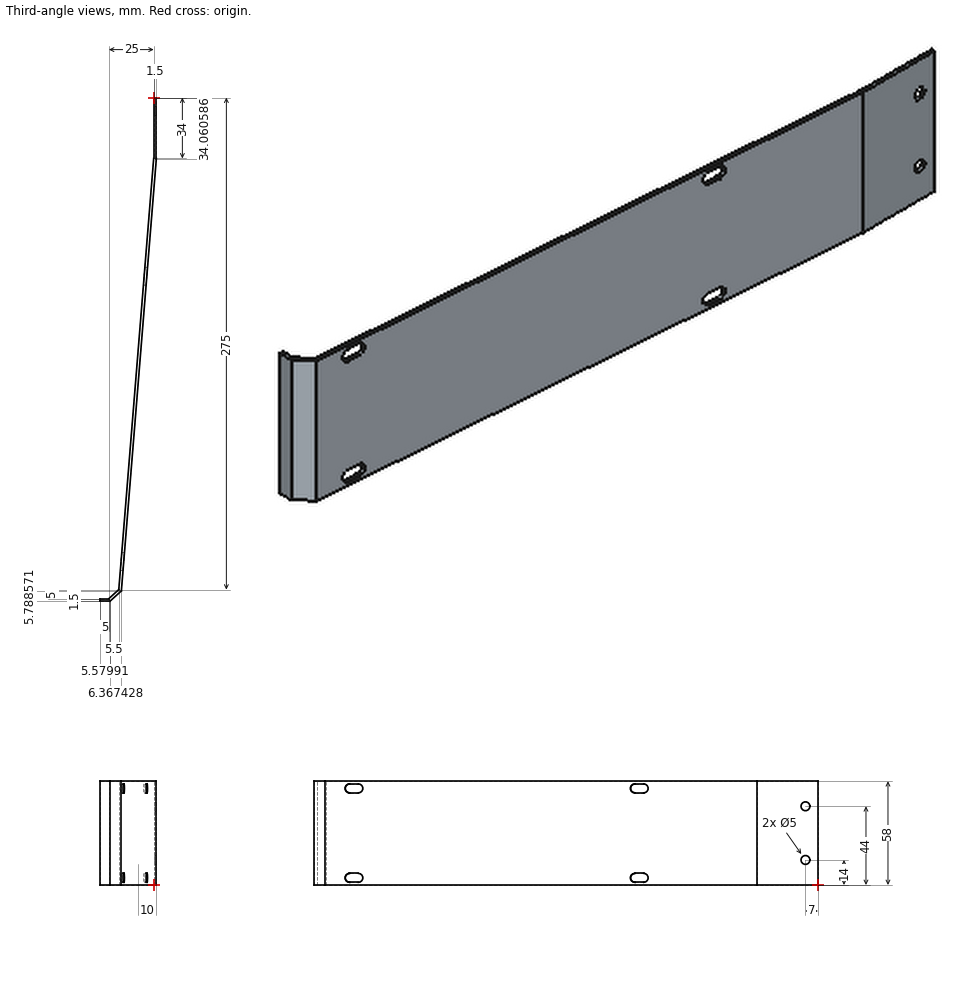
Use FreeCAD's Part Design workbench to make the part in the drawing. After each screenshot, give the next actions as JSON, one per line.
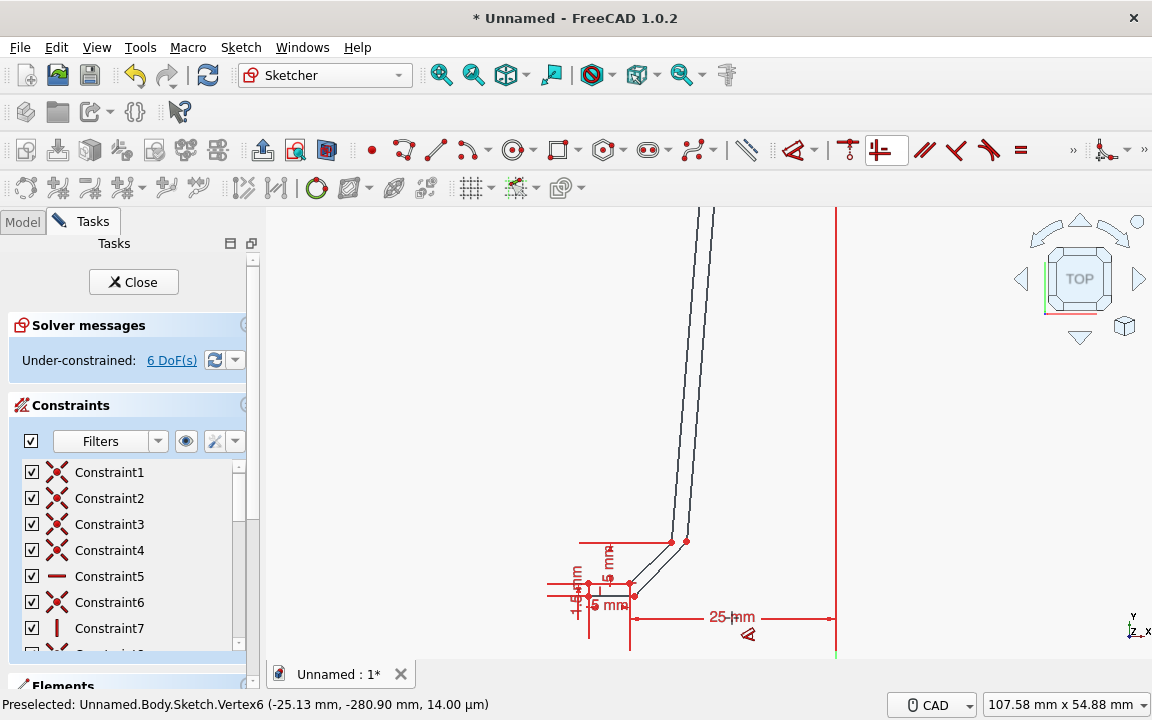
{"action": "left_click", "coordinate": [672, 543]}
{"action": "left_click", "coordinate": [870, 389]}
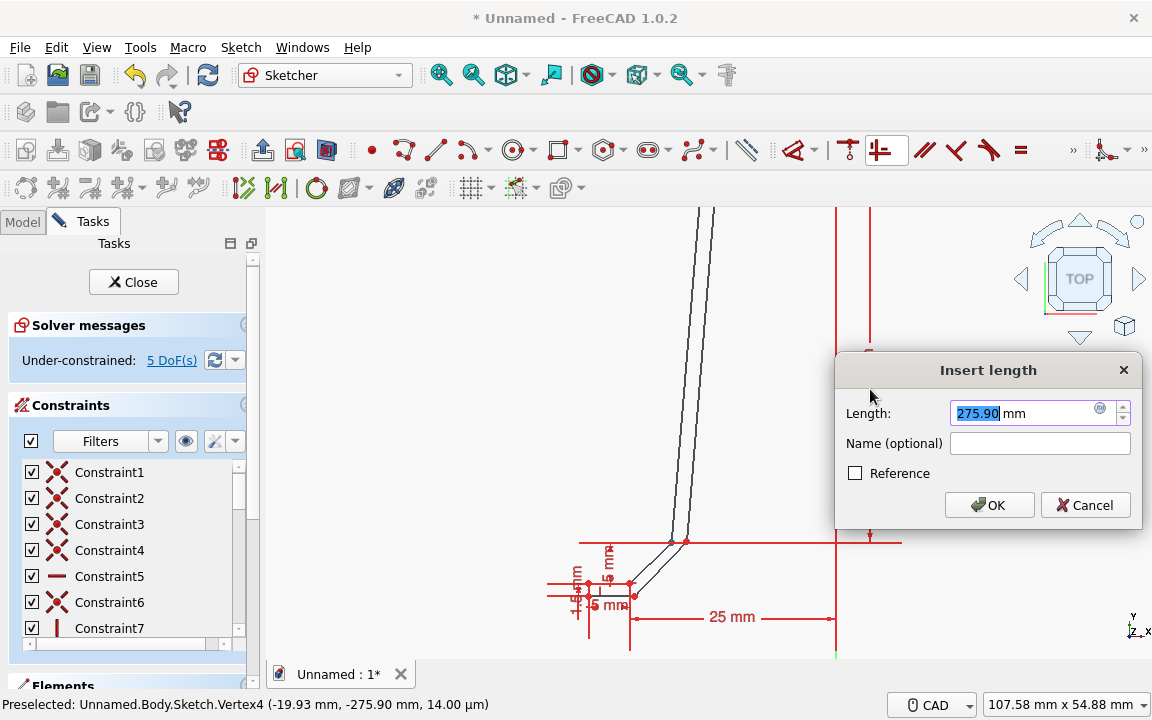
{"action": "type", "text": "275"}
{"action": "key", "text": "Return"}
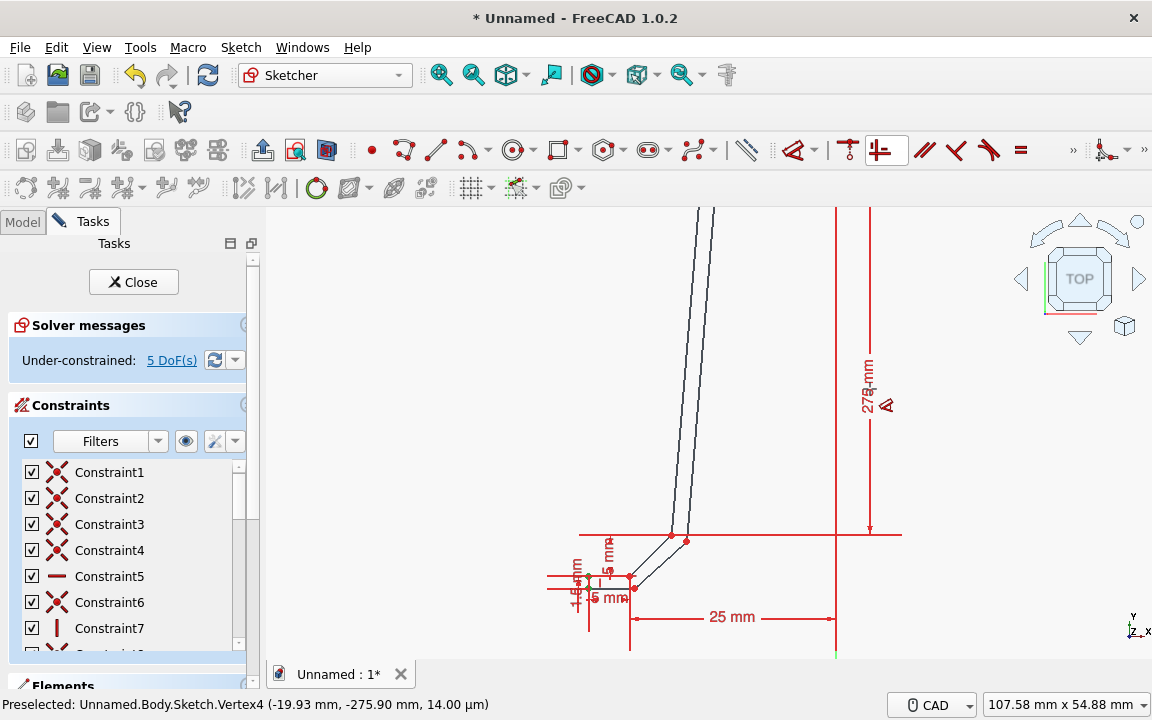
{"action": "left_click", "coordinate": [659, 548]}
{"action": "left_click", "coordinate": [651, 501]}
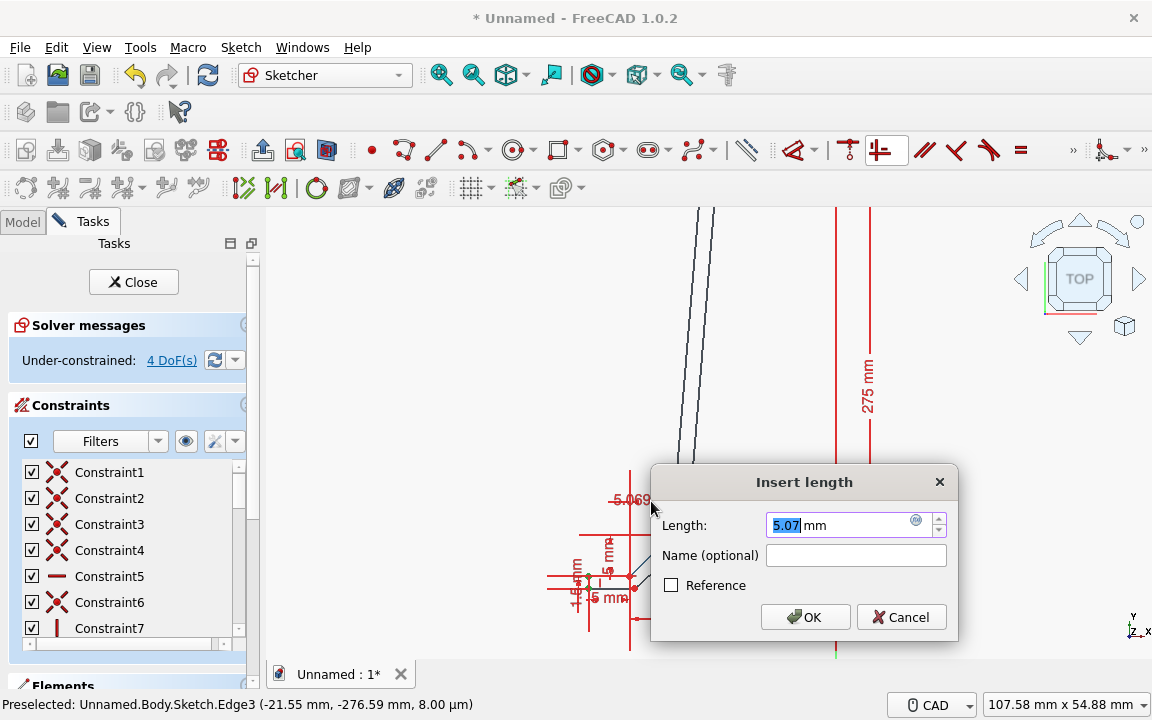
{"action": "type", "text": "5.5"}
{"action": "key", "text": "Return"}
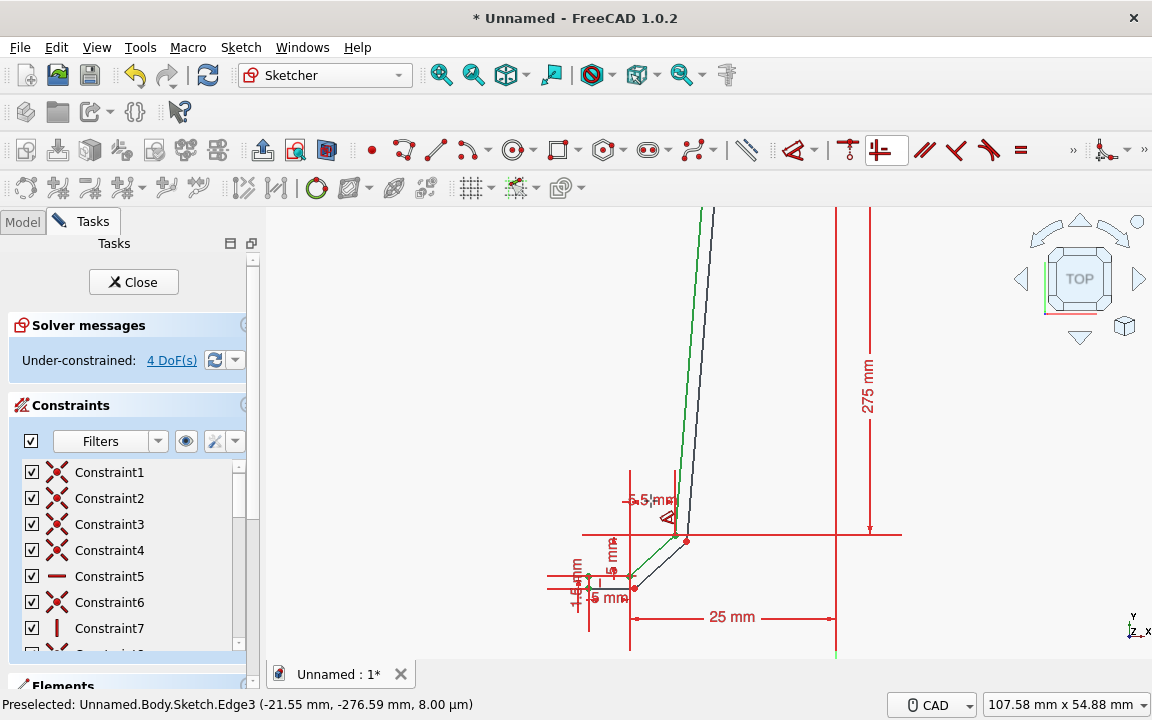
{"action": "left_click", "coordinate": [603, 589]}
{"action": "left_click", "coordinate": [612, 623]}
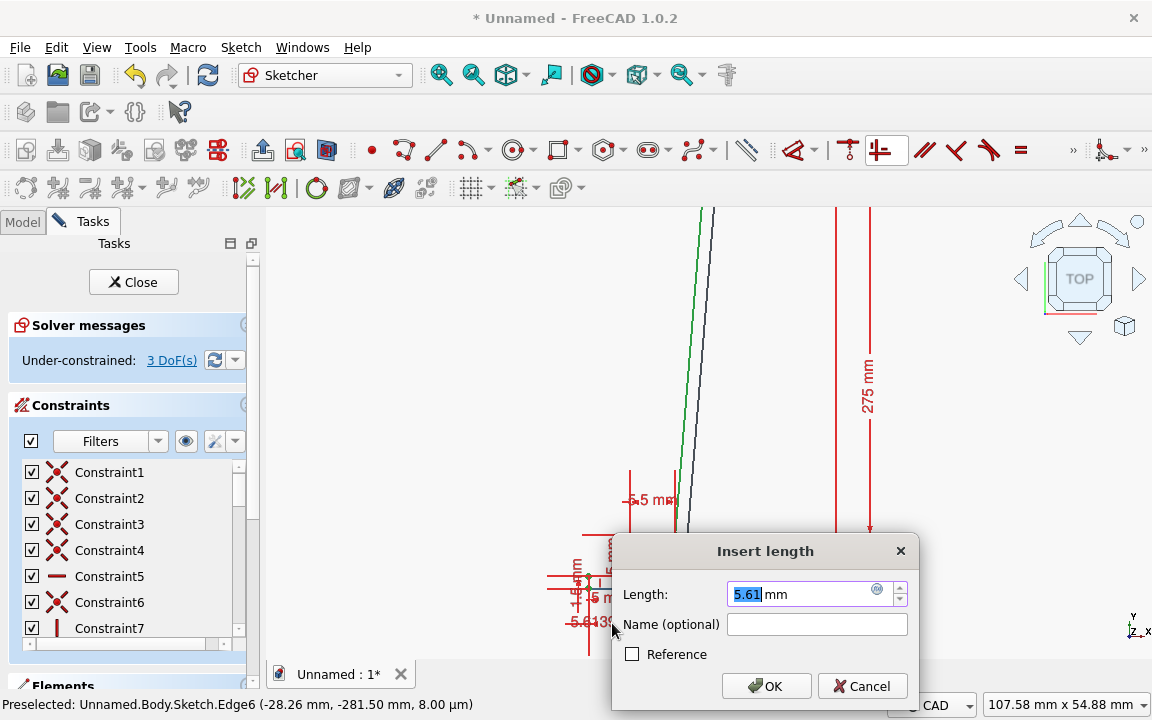
{"action": "type", "text": "5.57991"}
{"action": "key", "text": "Return"}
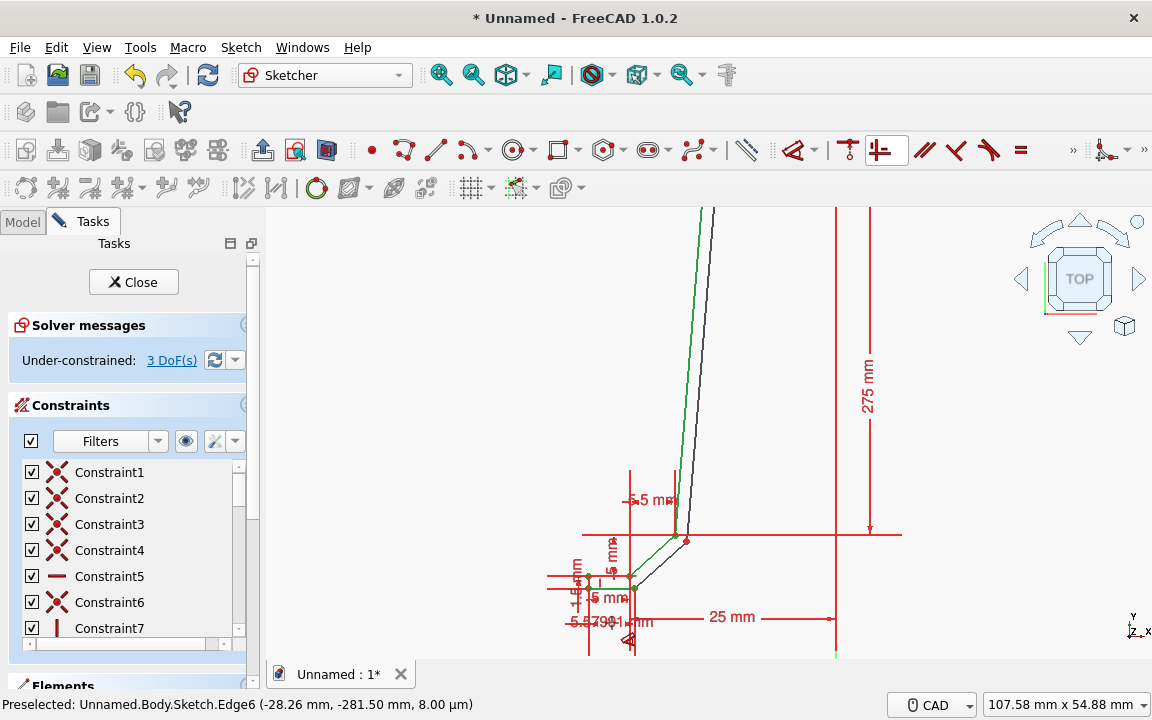
{"action": "scroll", "coordinate": [631, 558], "scroll_direction": "down", "scroll_amount": 11}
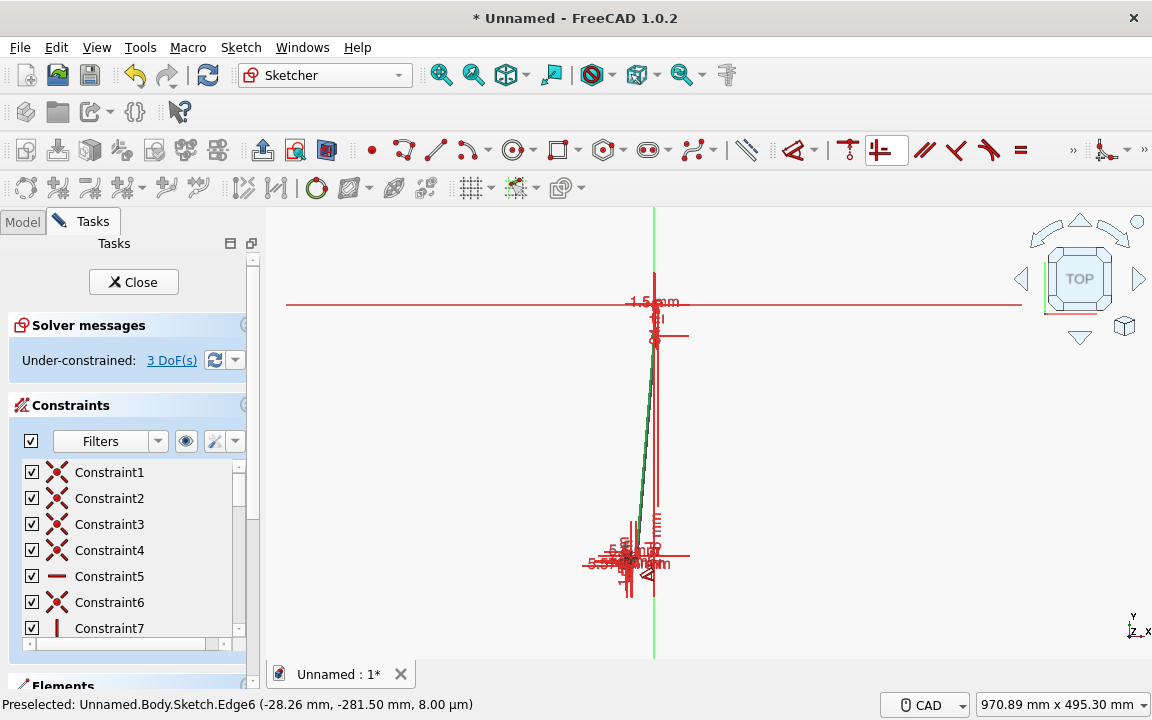
{"action": "scroll", "coordinate": [655, 327], "scroll_direction": "up", "scroll_amount": 12}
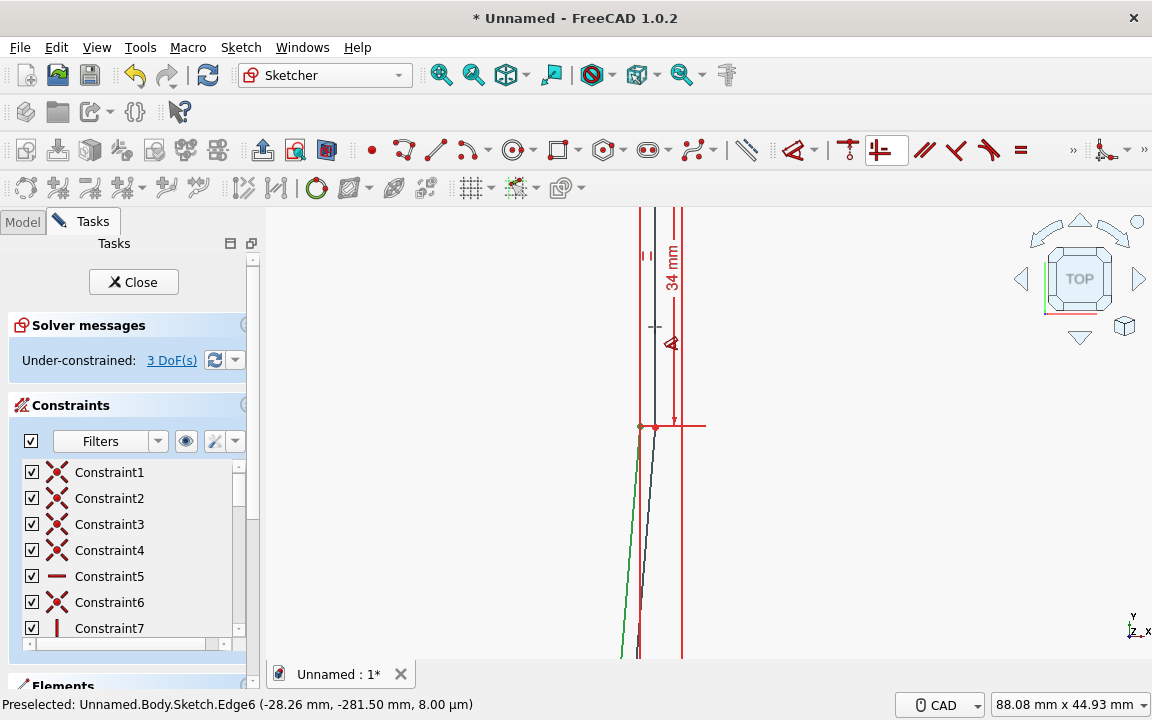
{"action": "left_click", "coordinate": [655, 325]}
{"action": "left_click", "coordinate": [689, 331]}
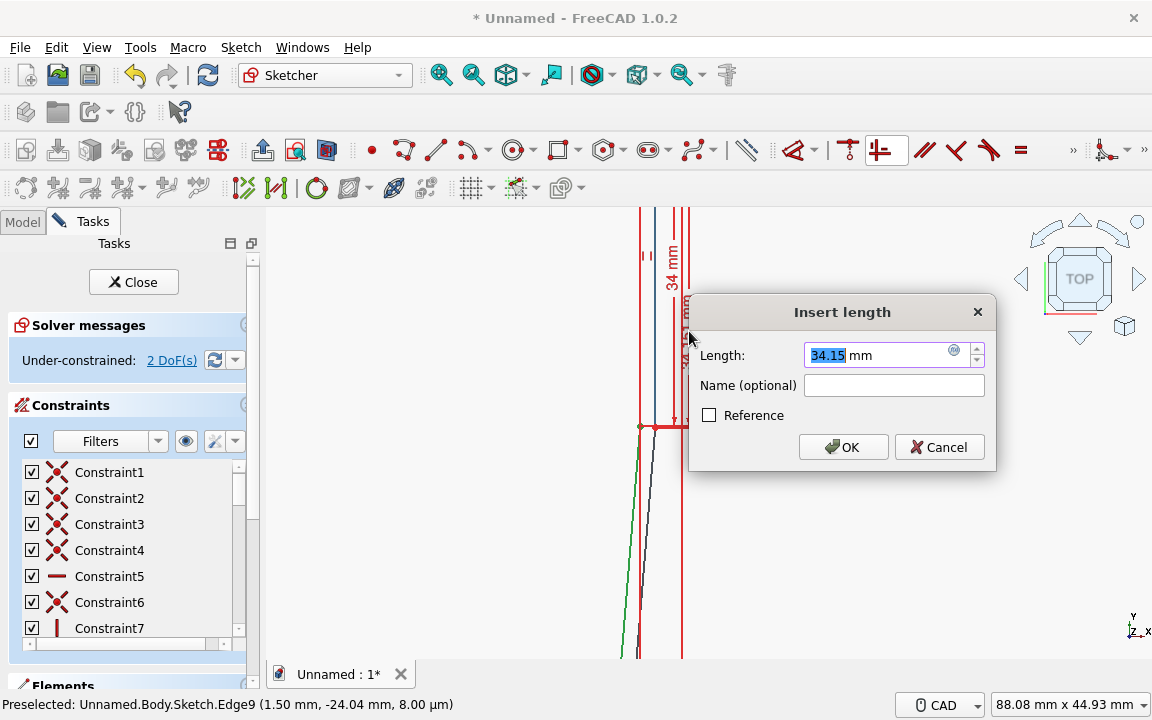
{"action": "type", "text": "34.060586"}
{"action": "key", "text": "Return"}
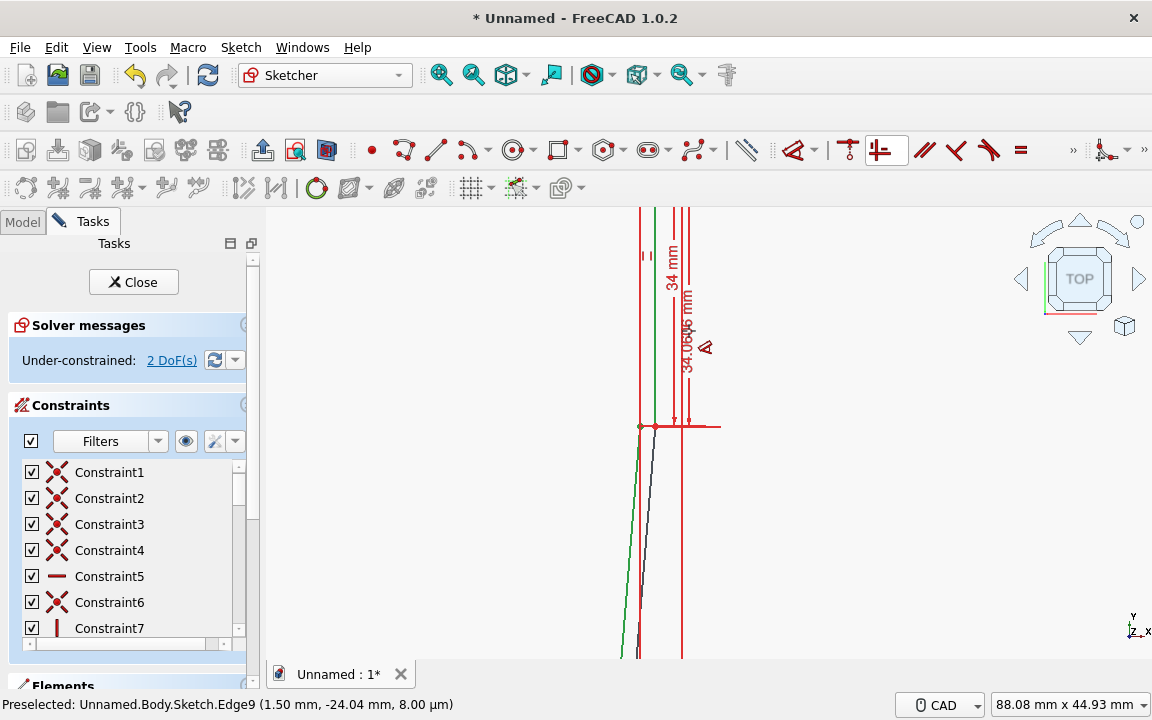
{"action": "scroll", "coordinate": [655, 327], "scroll_direction": "down", "scroll_amount": 12}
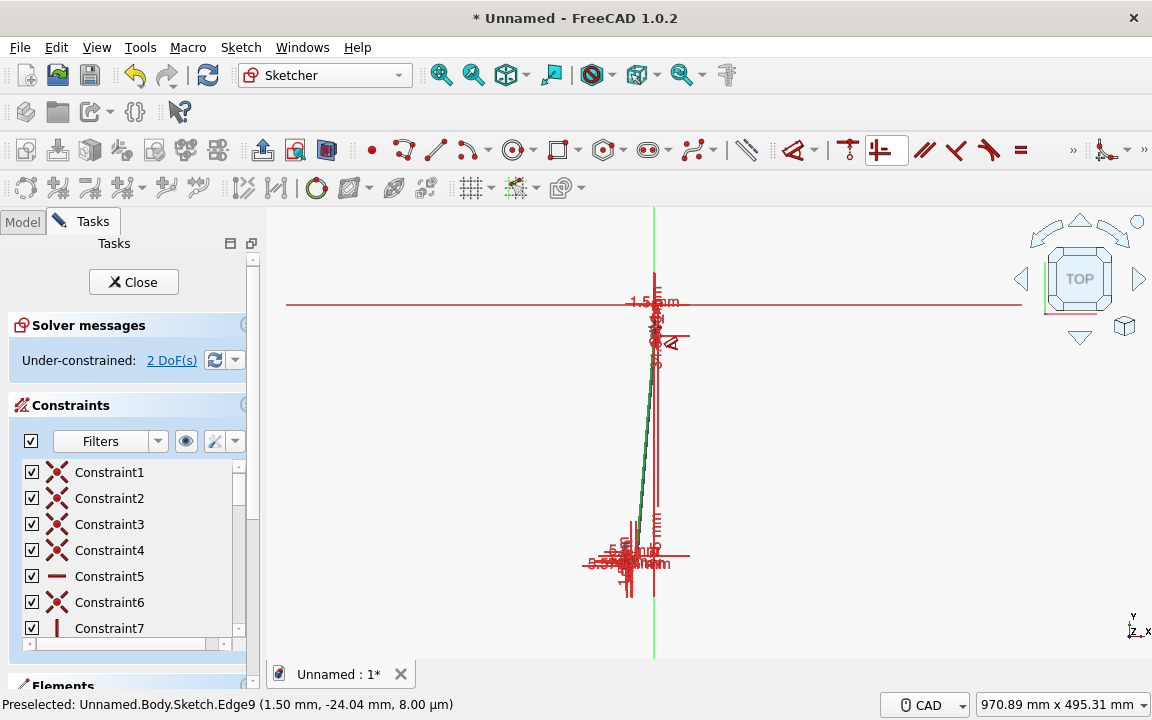
{"action": "scroll", "coordinate": [634, 561], "scroll_direction": "up", "scroll_amount": 12}